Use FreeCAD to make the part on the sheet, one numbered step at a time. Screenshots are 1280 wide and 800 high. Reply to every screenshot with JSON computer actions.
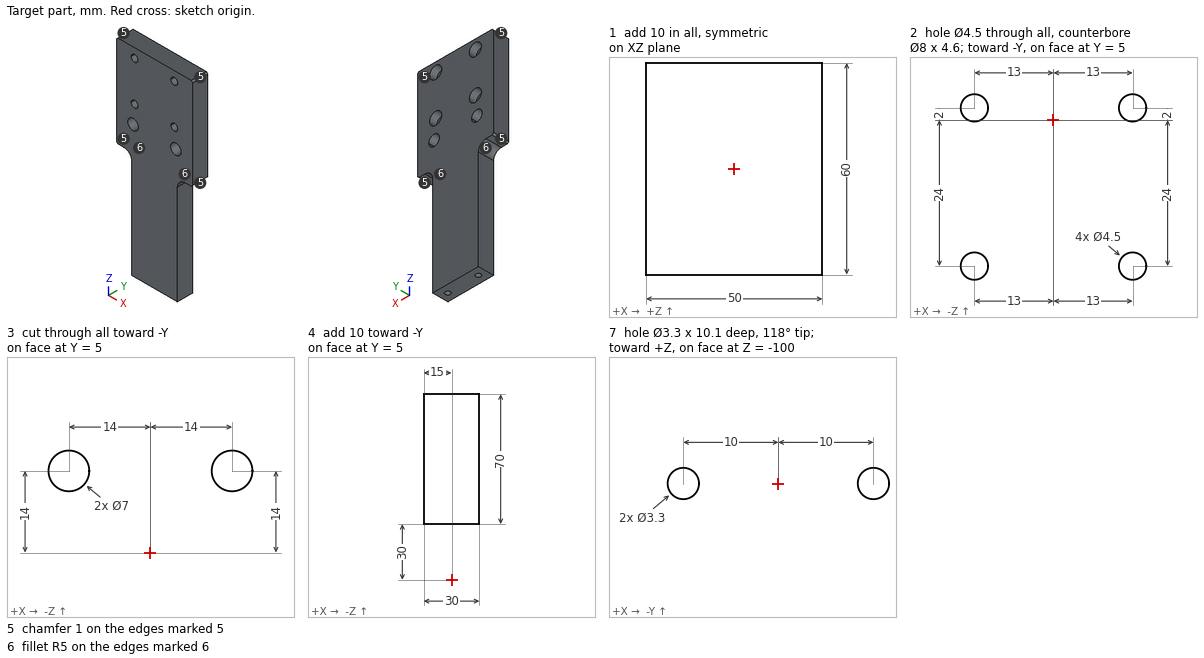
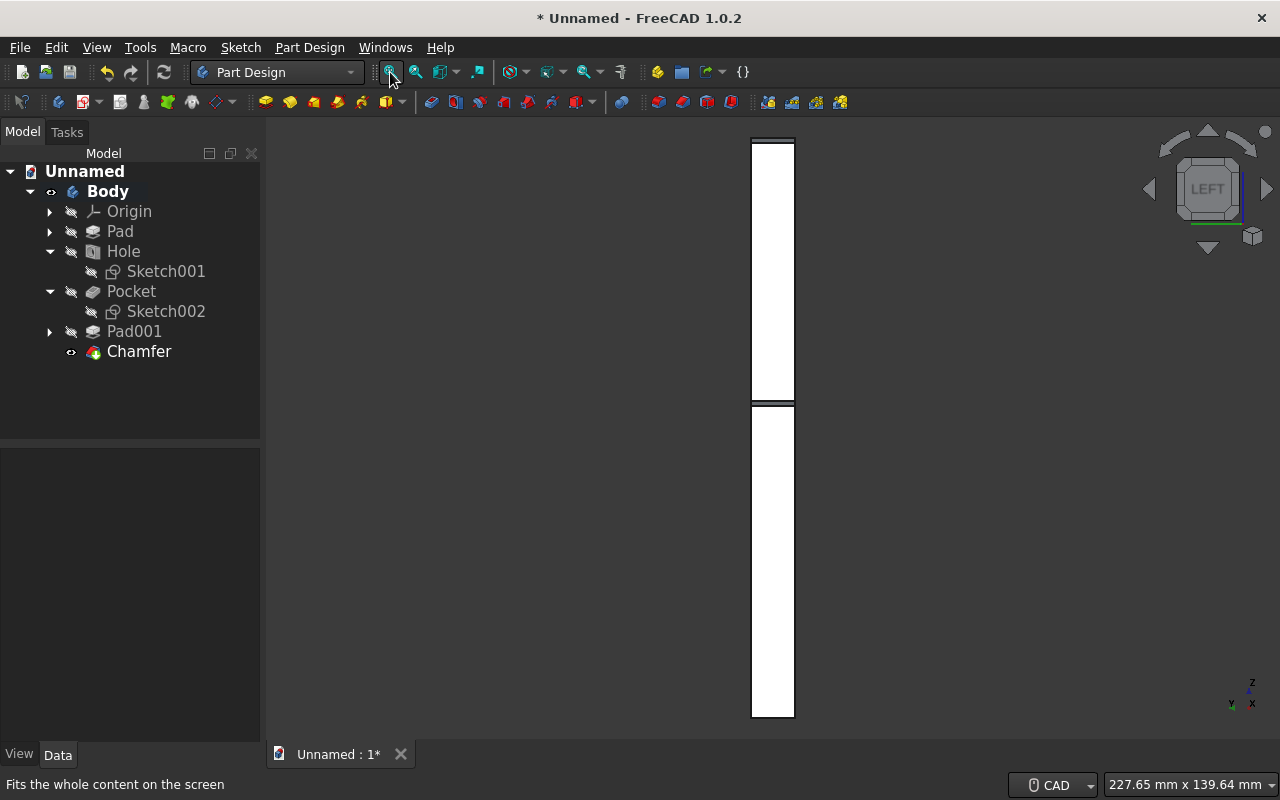
{"action": "key", "text": "v 3"}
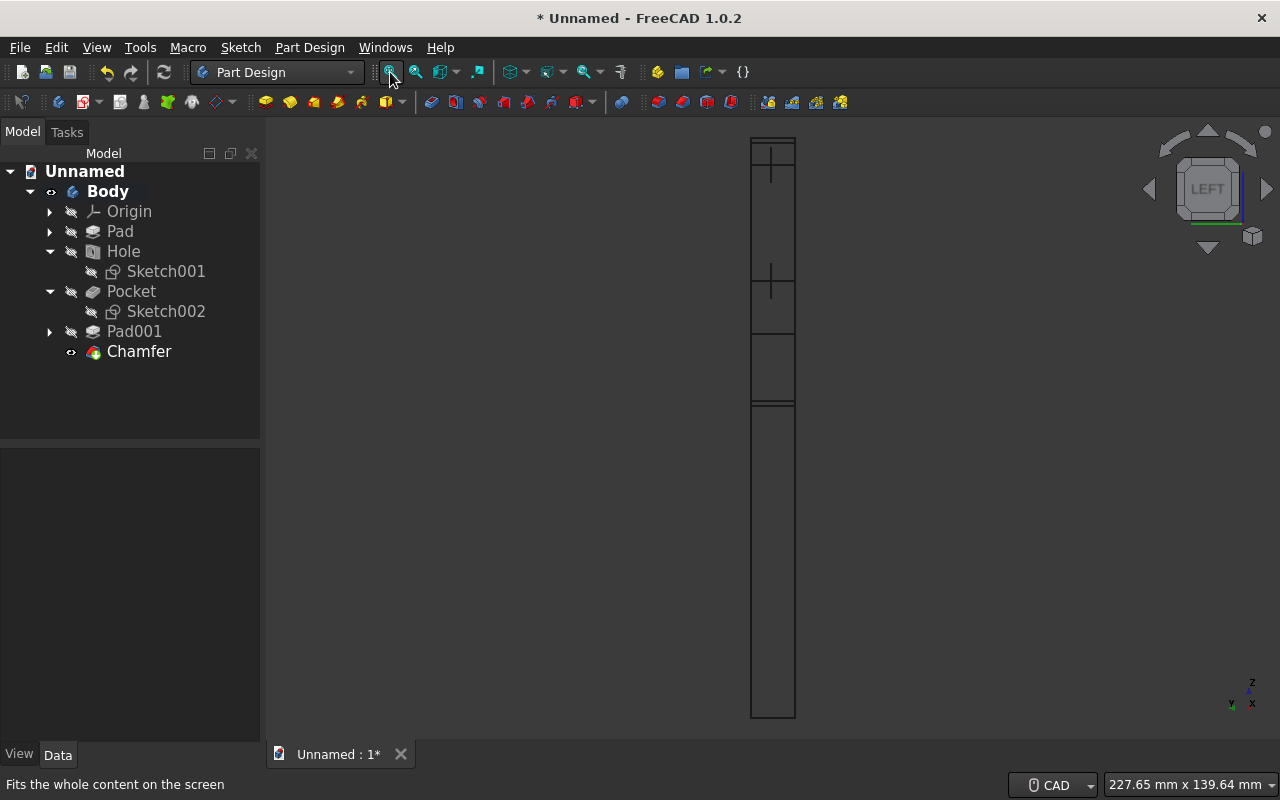
{"action": "key", "text": "0"}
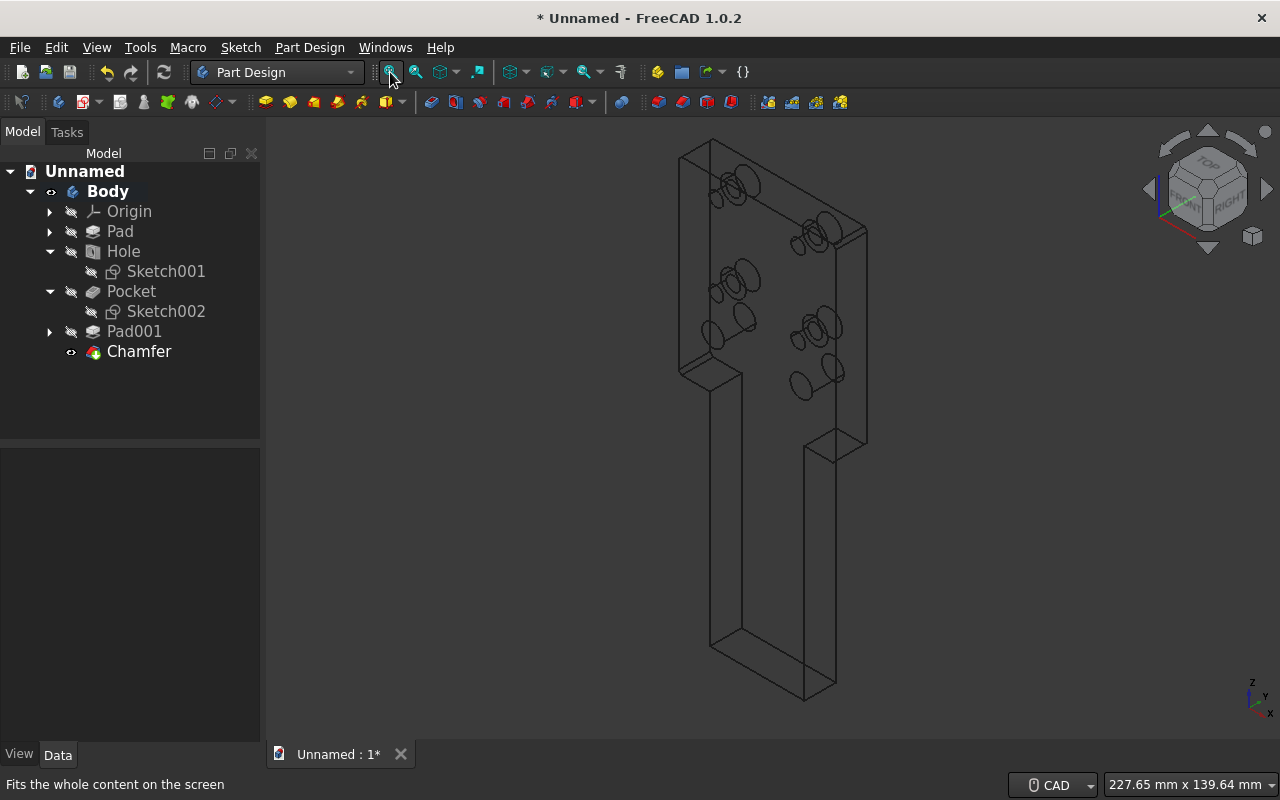
{"action": "left_click", "coordinate": [726, 382]}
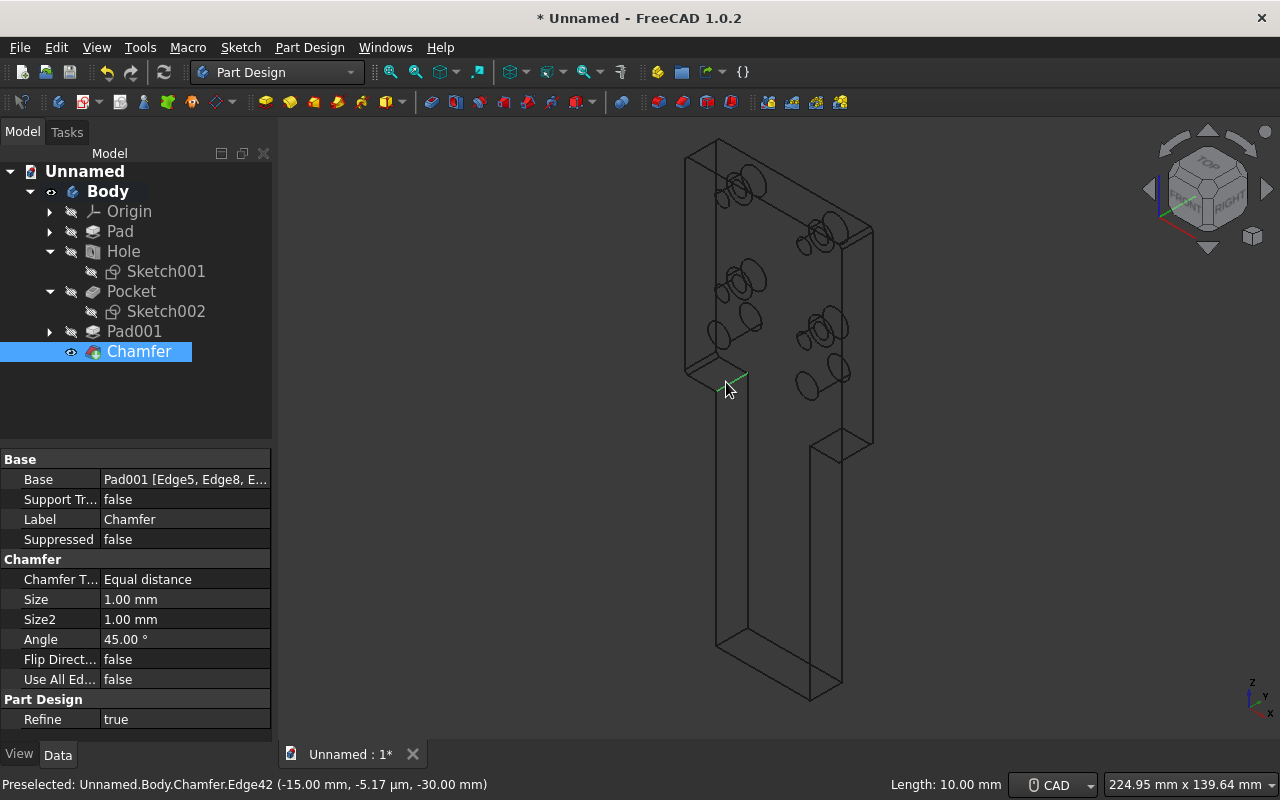
{"action": "left_click", "coordinate": [826, 436], "text": "ctrl"}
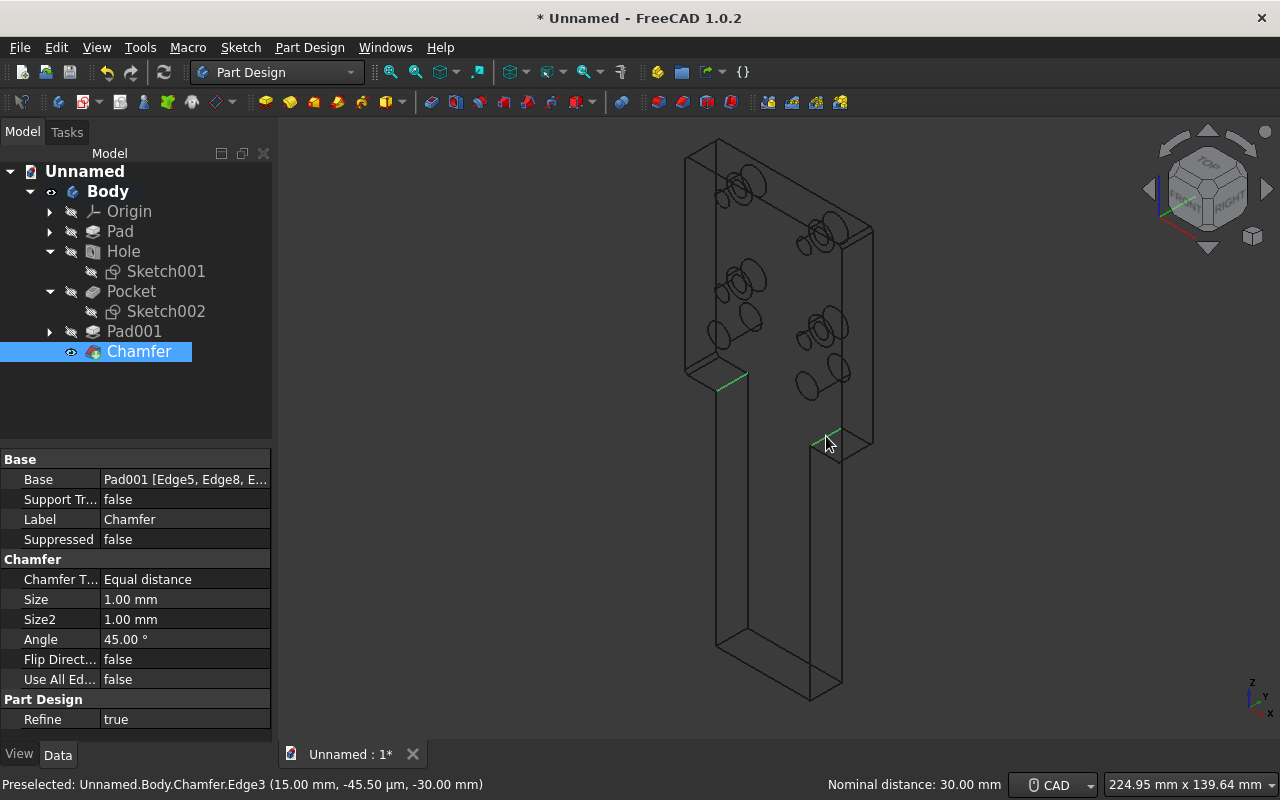
{"action": "key", "text": "v 1"}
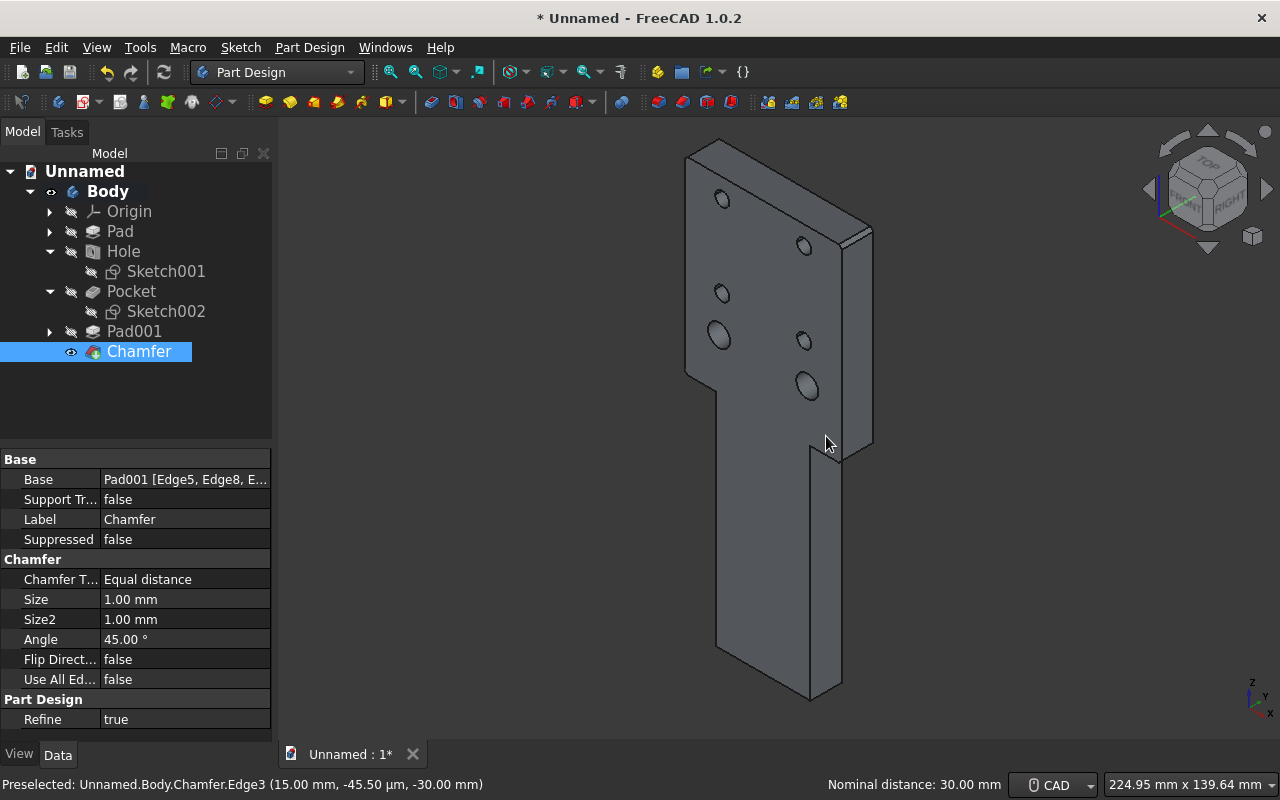
{"action": "left_click", "coordinate": [660, 102]}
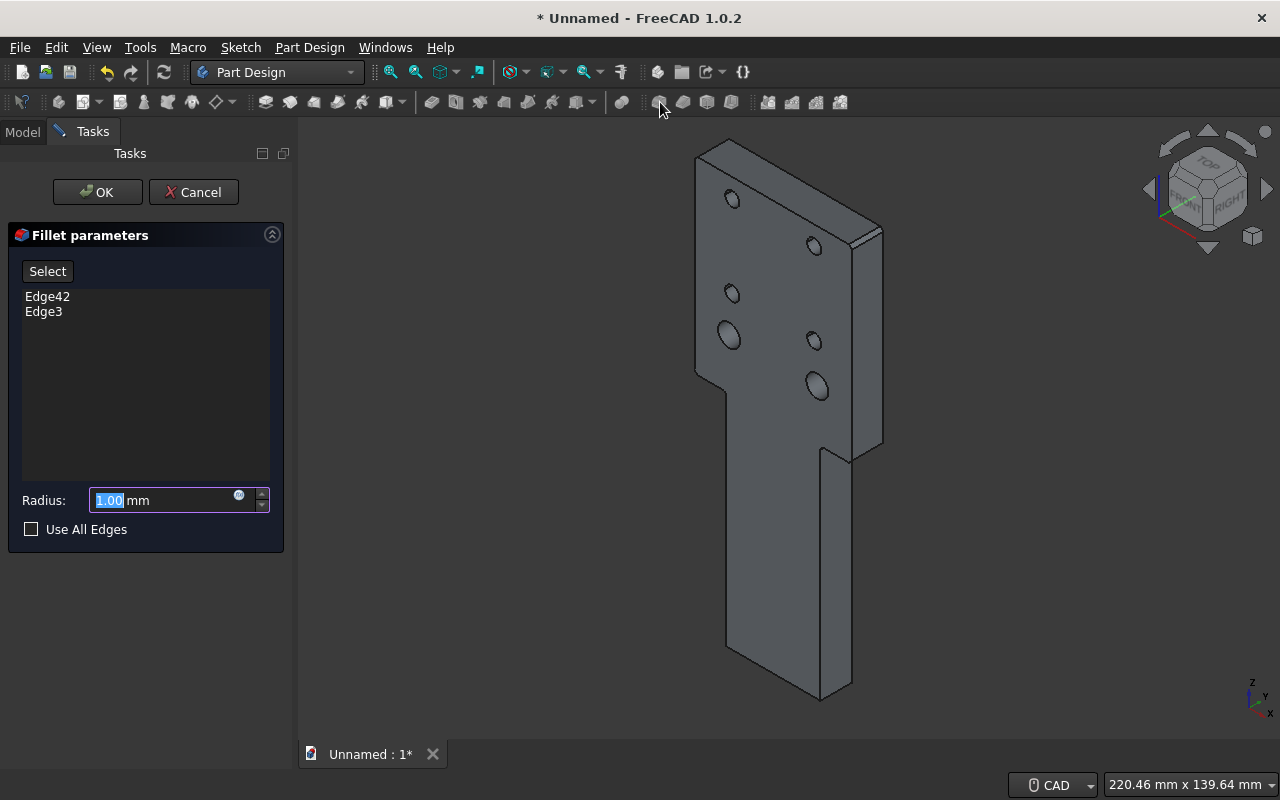
{"action": "type", "text": "5"}
{"action": "key", "text": "Tab"}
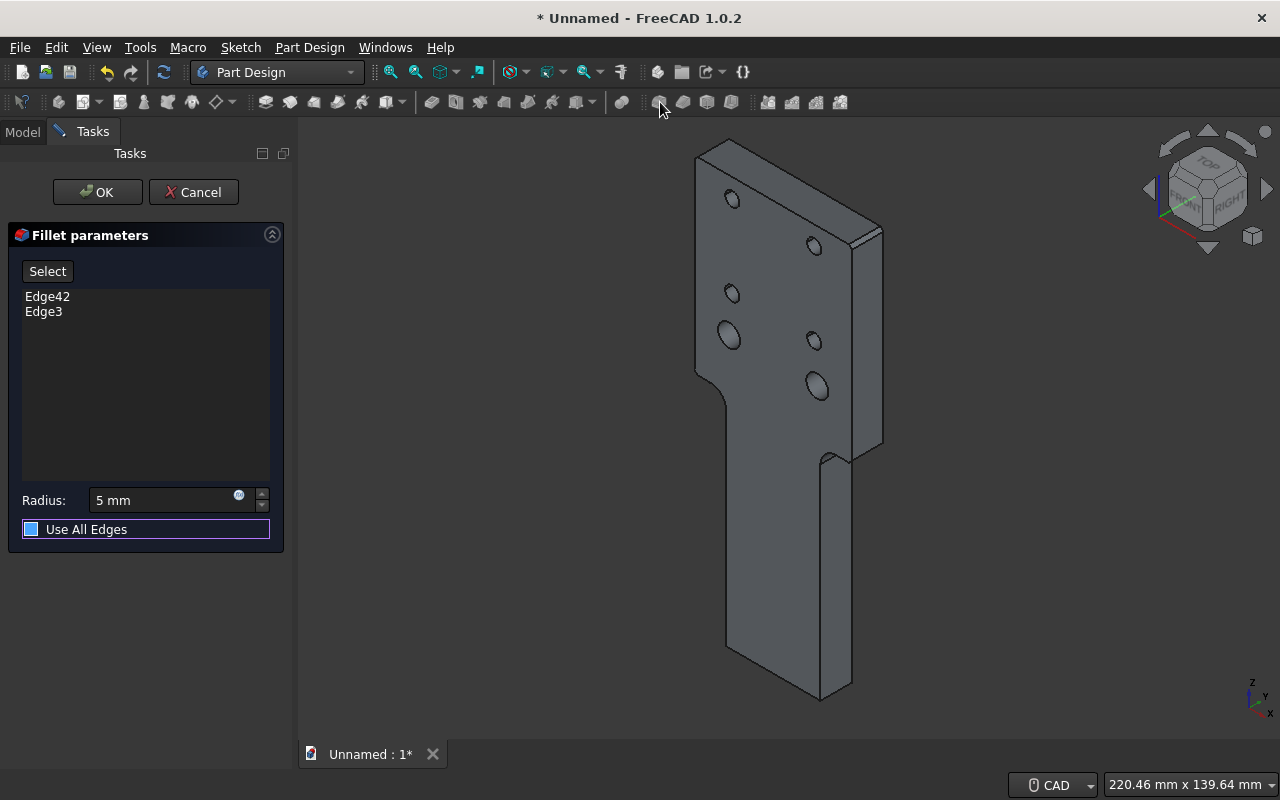
{"action": "left_click", "coordinate": [98, 192]}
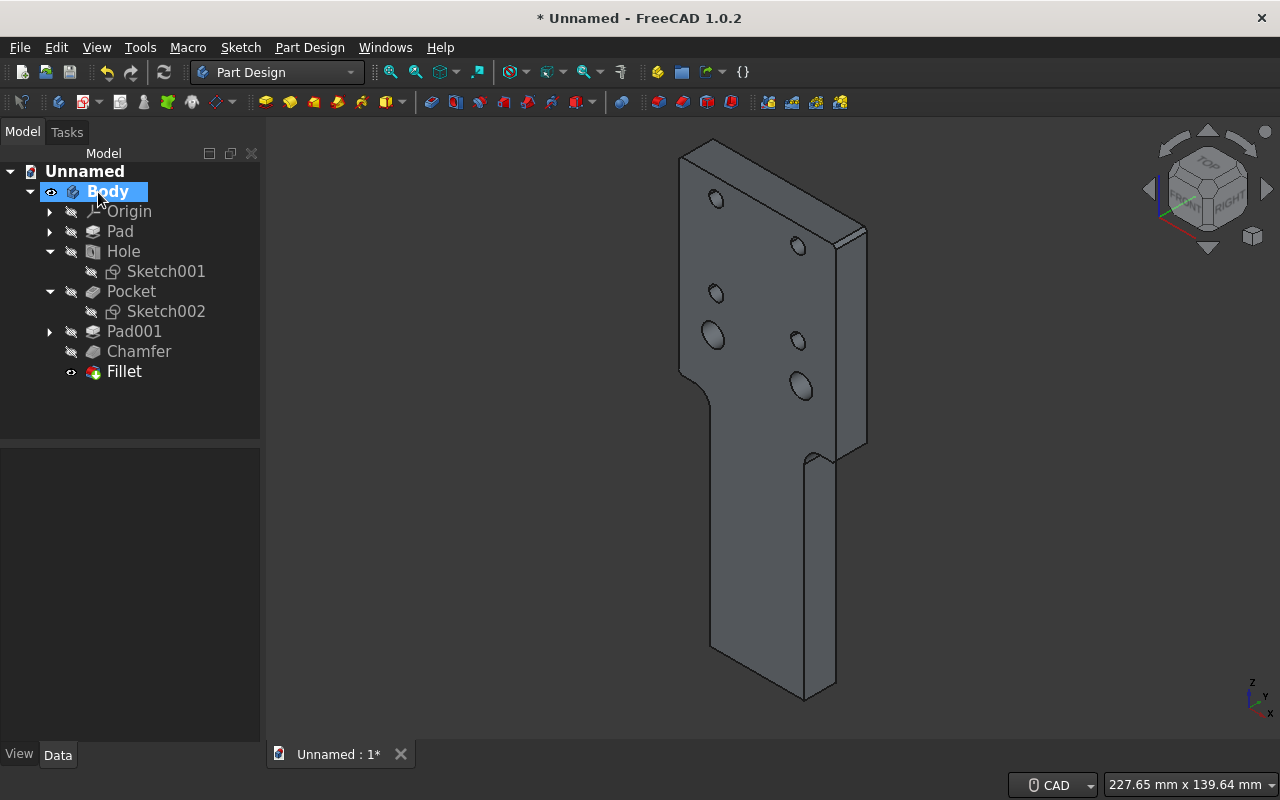
{"action": "key", "text": "5"}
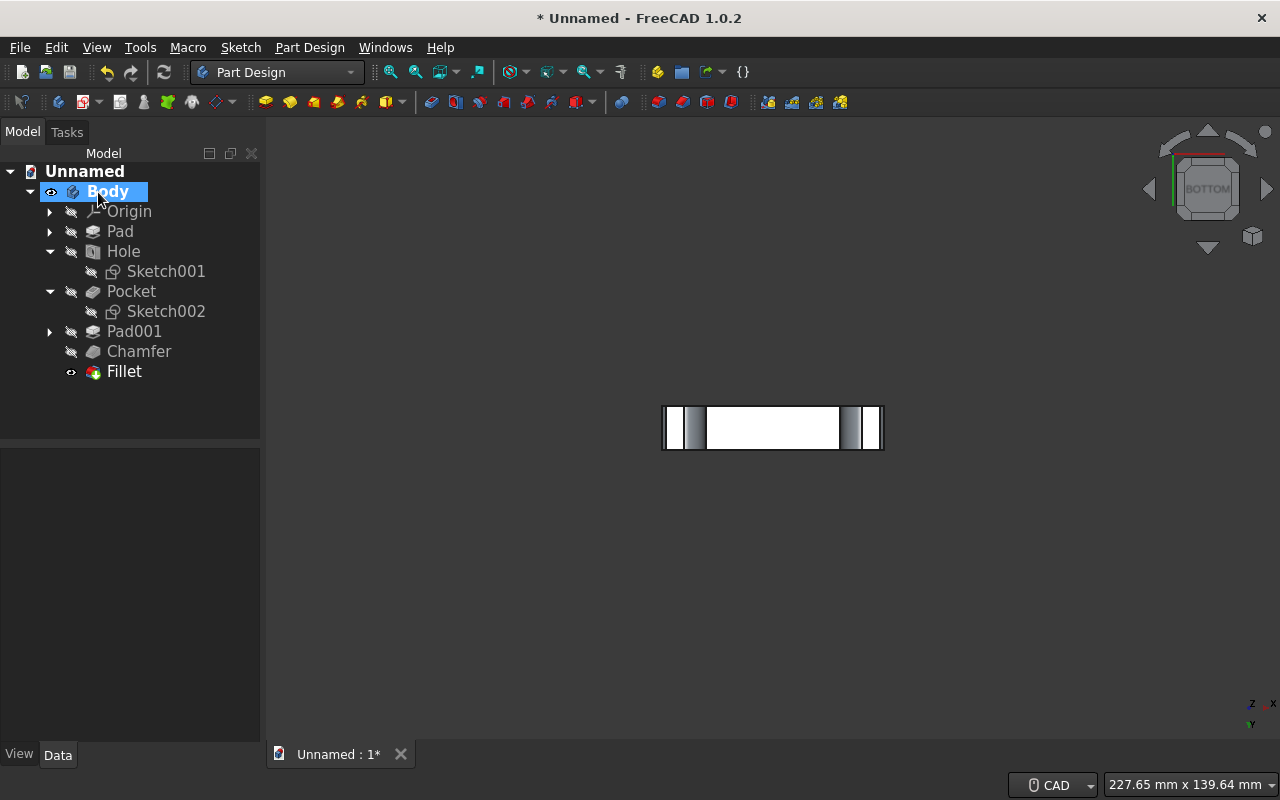
{"action": "left_click", "coordinate": [392, 72]}